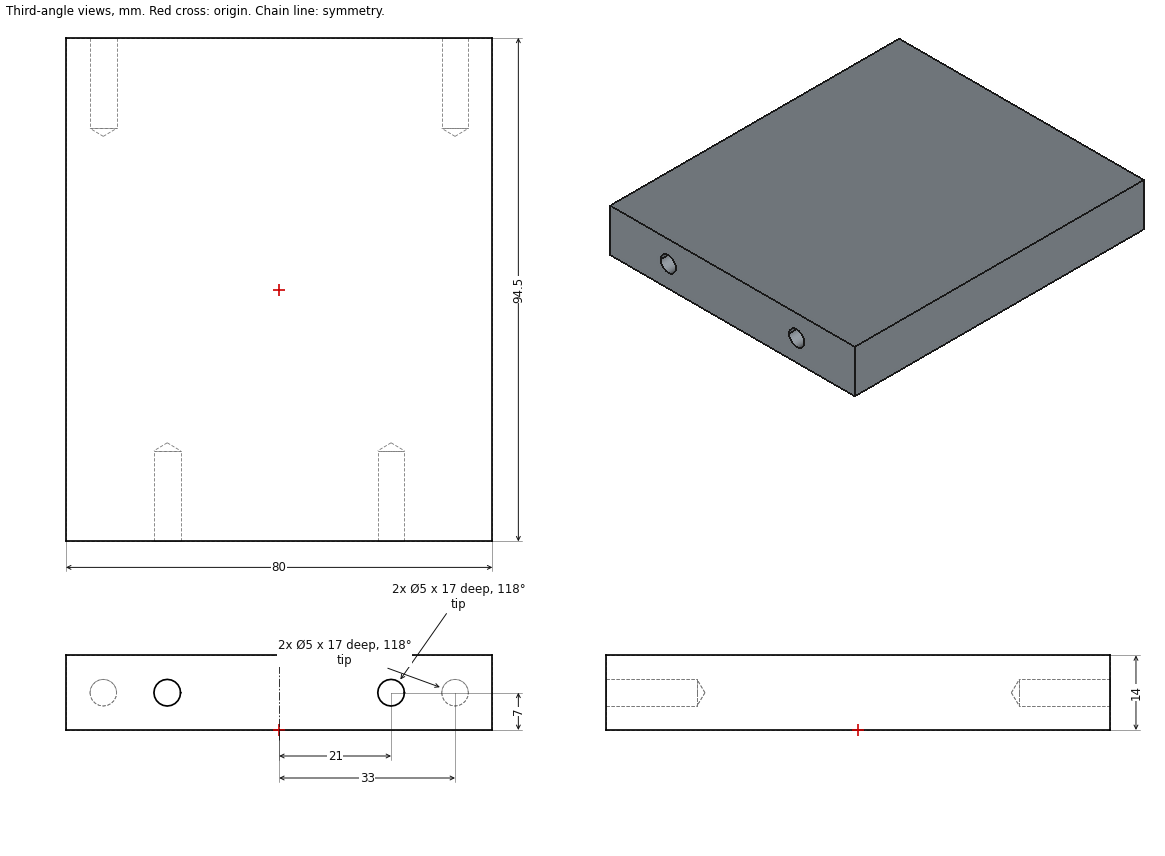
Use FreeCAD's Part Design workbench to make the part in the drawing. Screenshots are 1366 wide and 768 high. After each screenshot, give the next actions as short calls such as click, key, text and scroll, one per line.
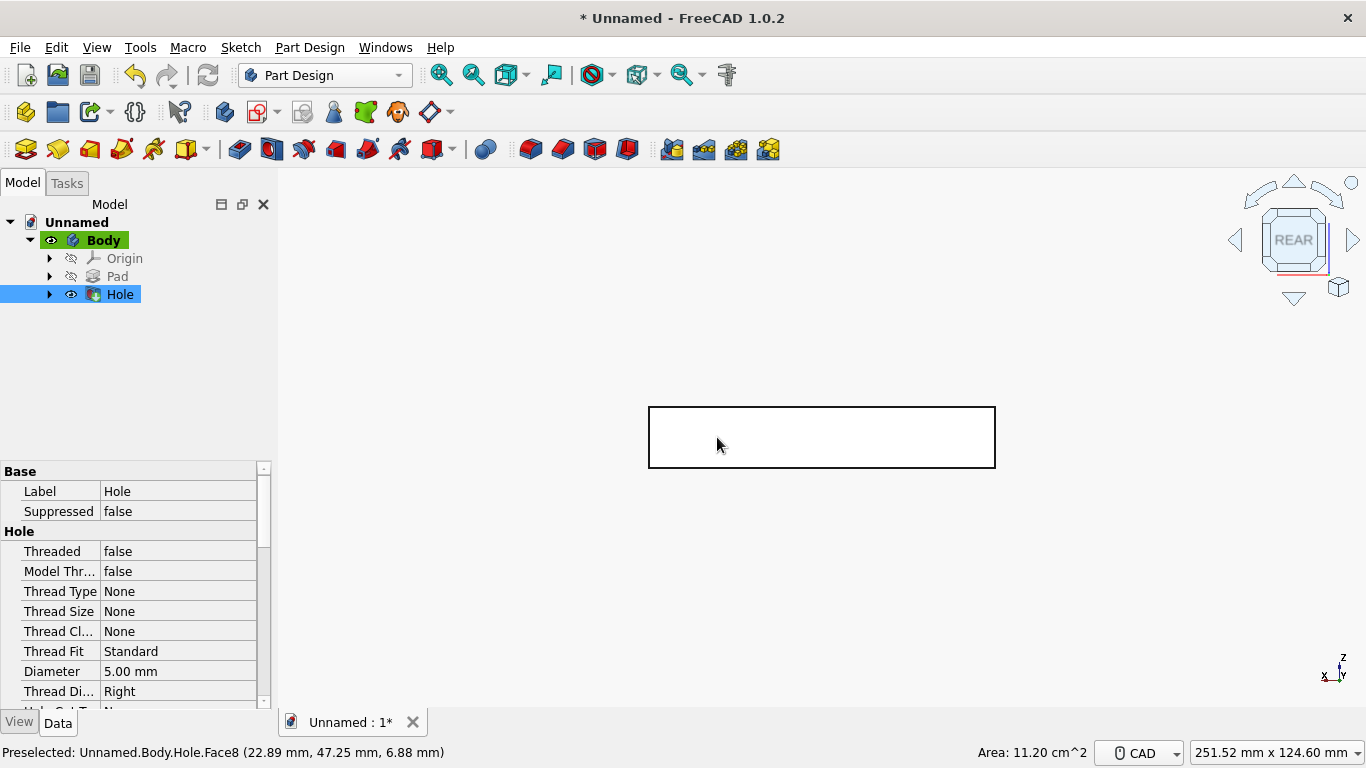
click(258, 112)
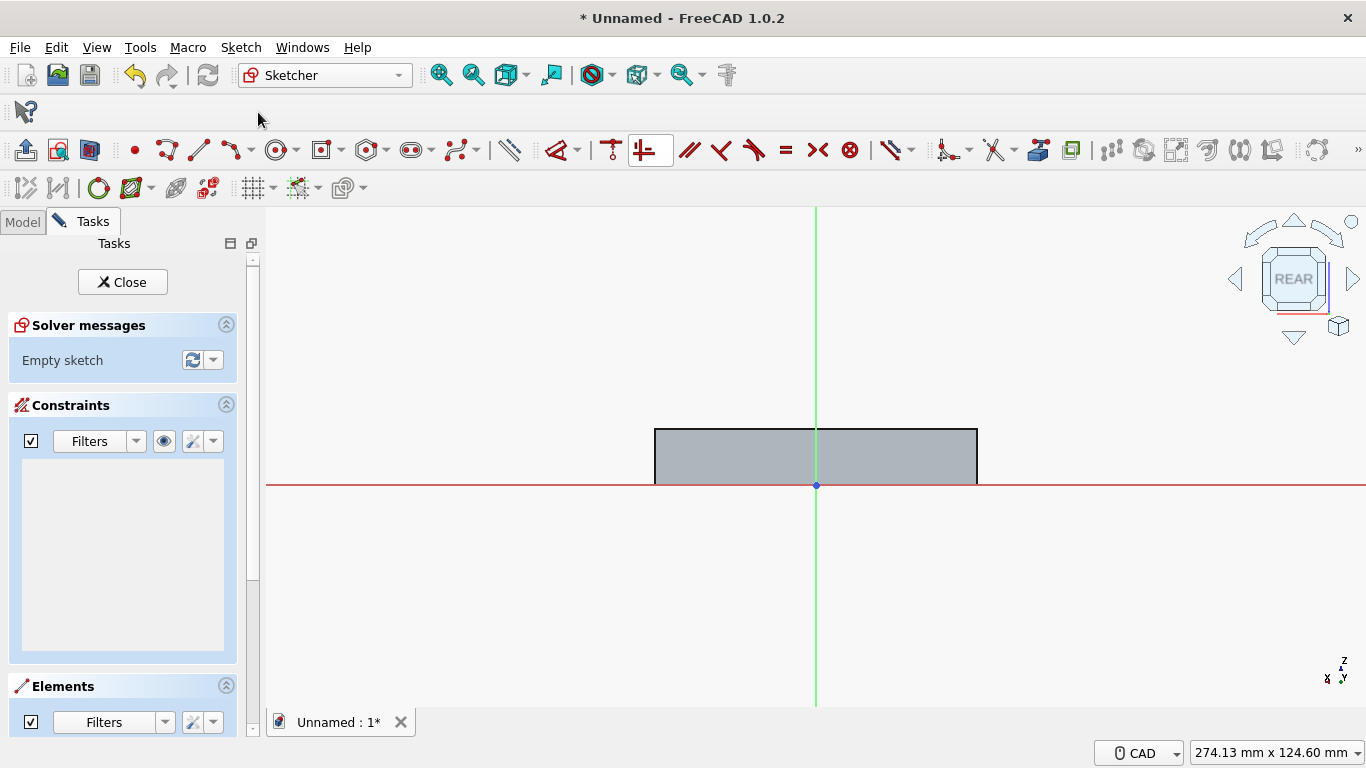
scroll(872, 473, up, 4)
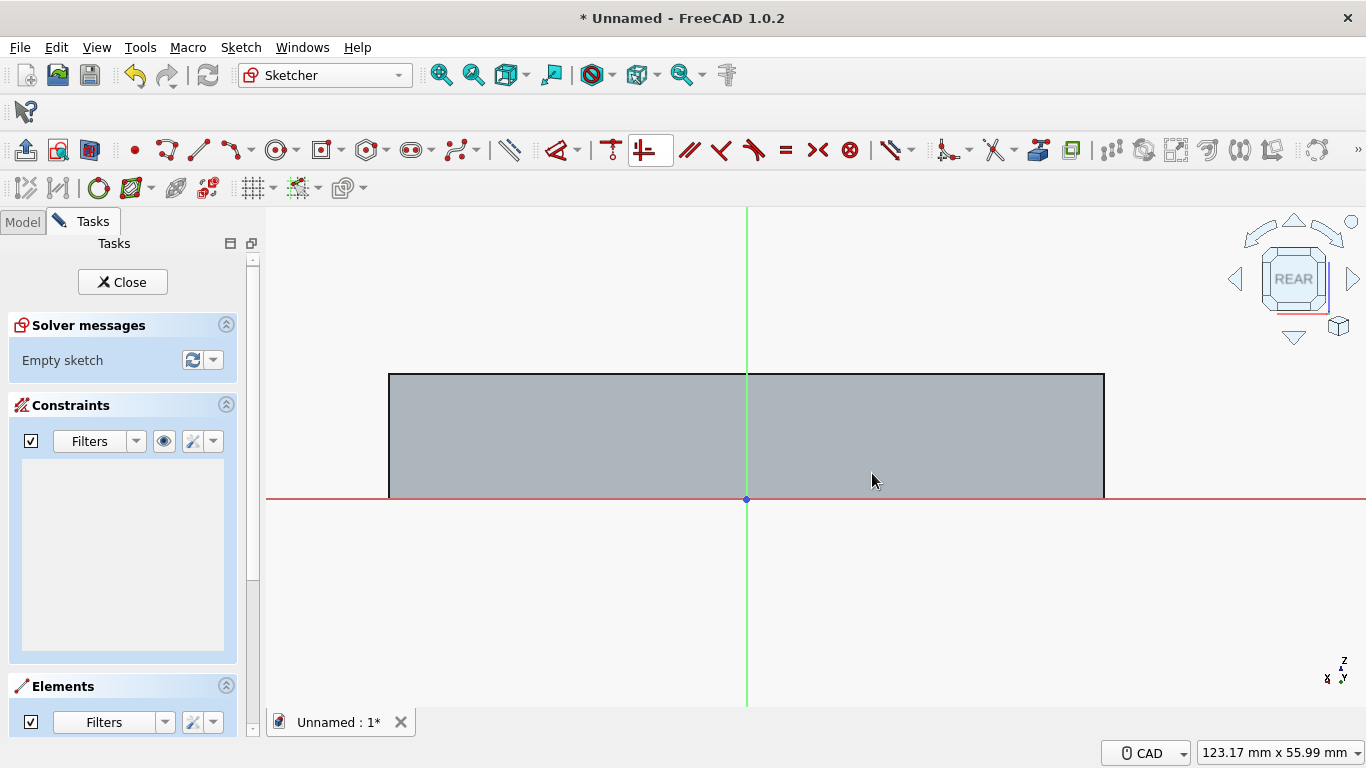
key(g)
key(c)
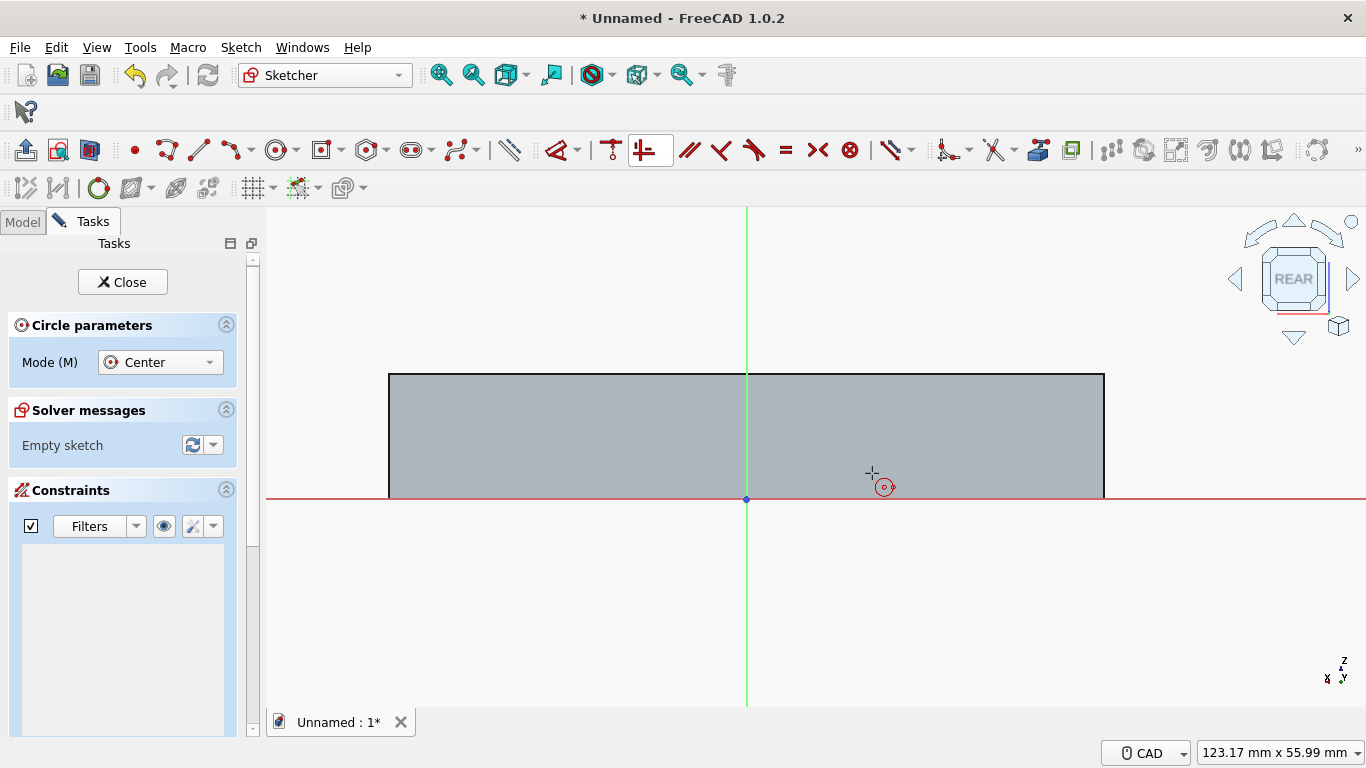
click(452, 437)
click(468, 421)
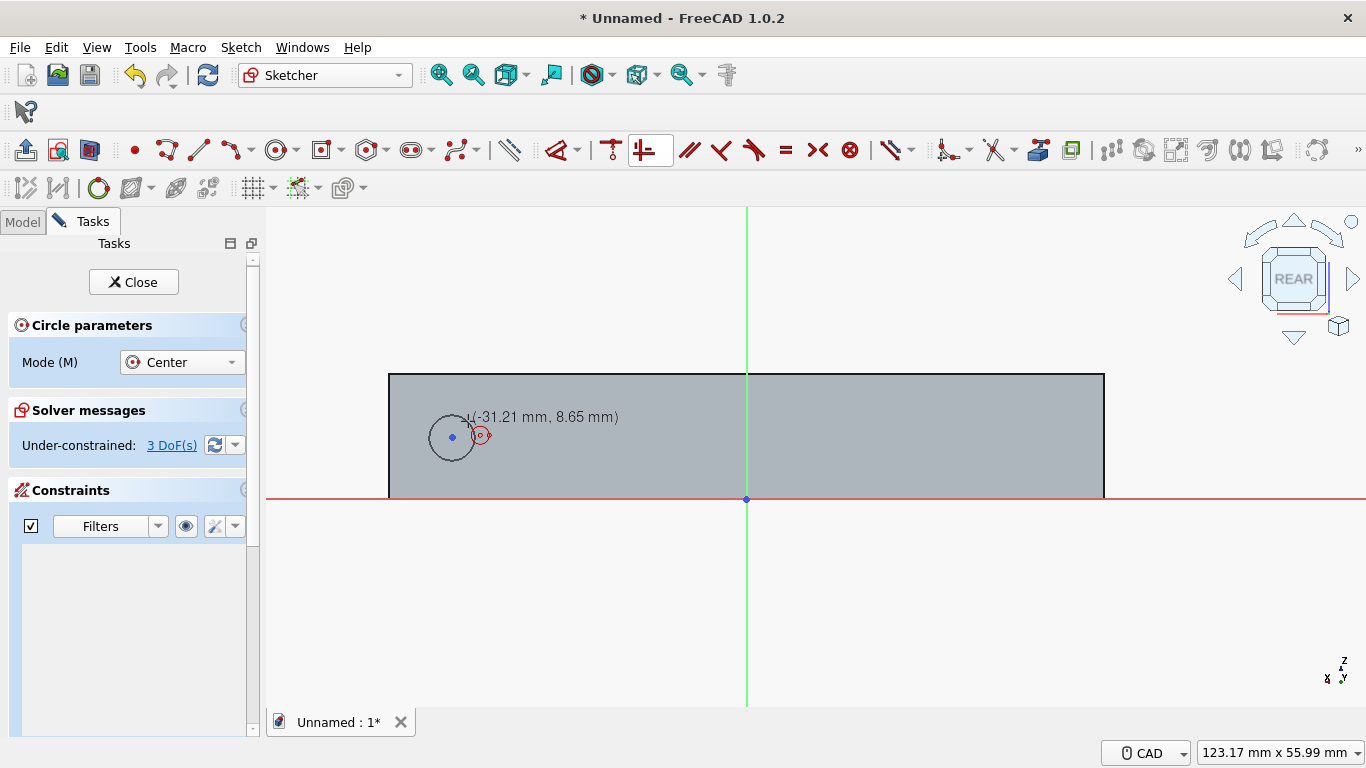
click(1041, 437)
click(1057, 421)
key(Escape)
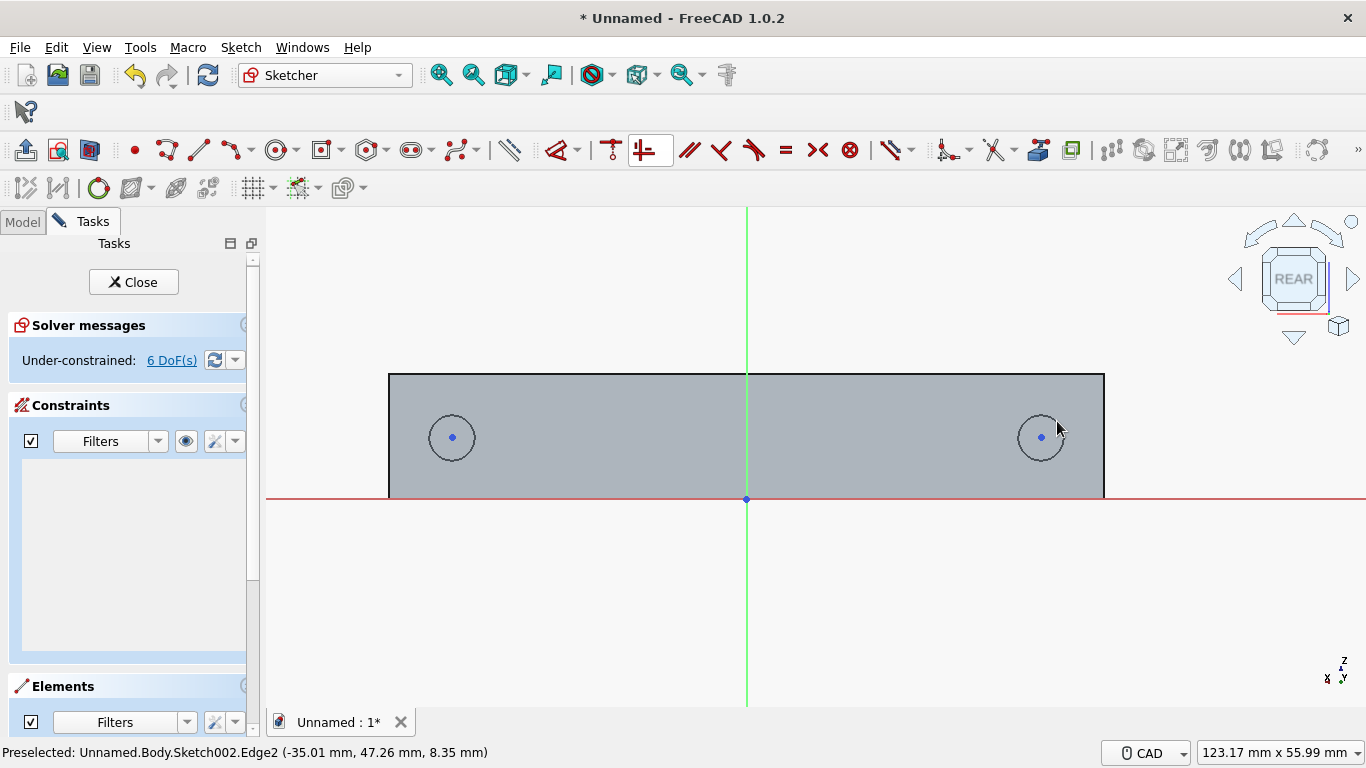
click(468, 422)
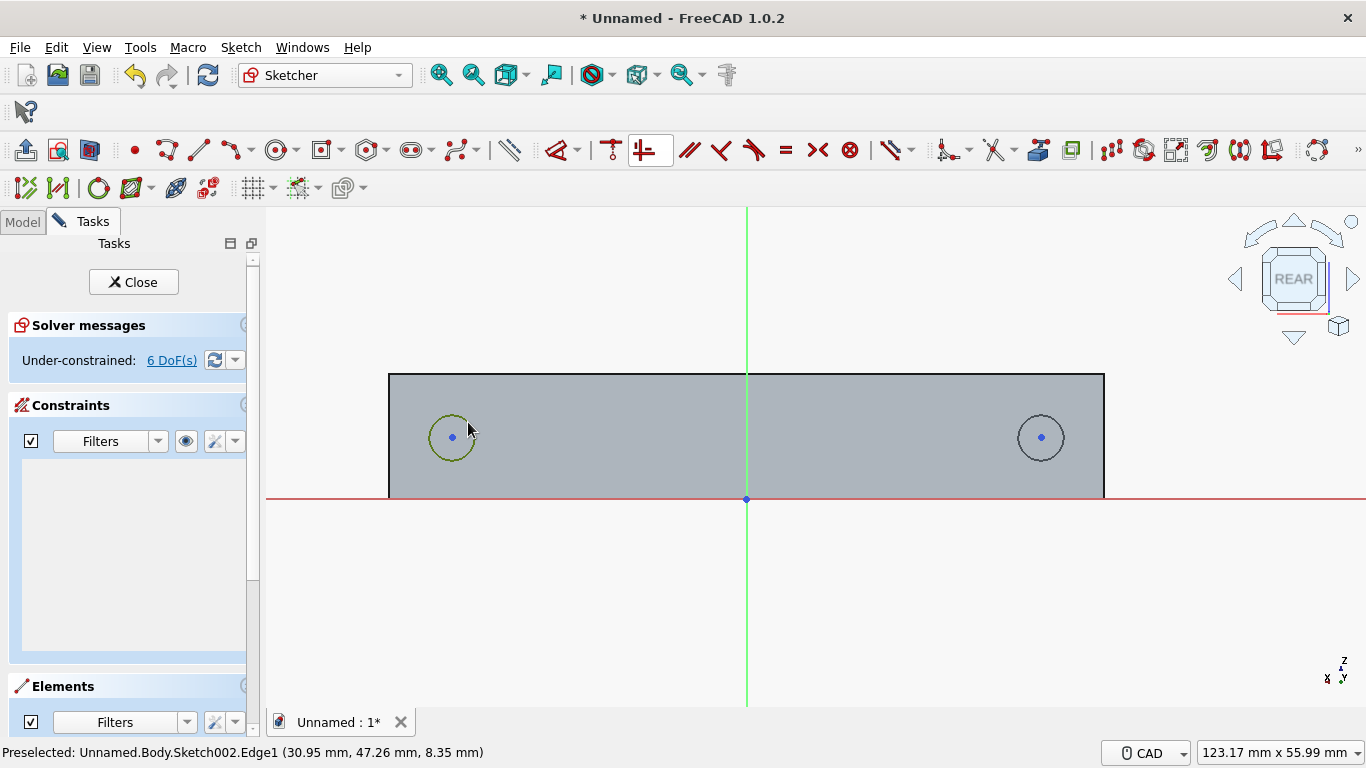
click(1057, 422)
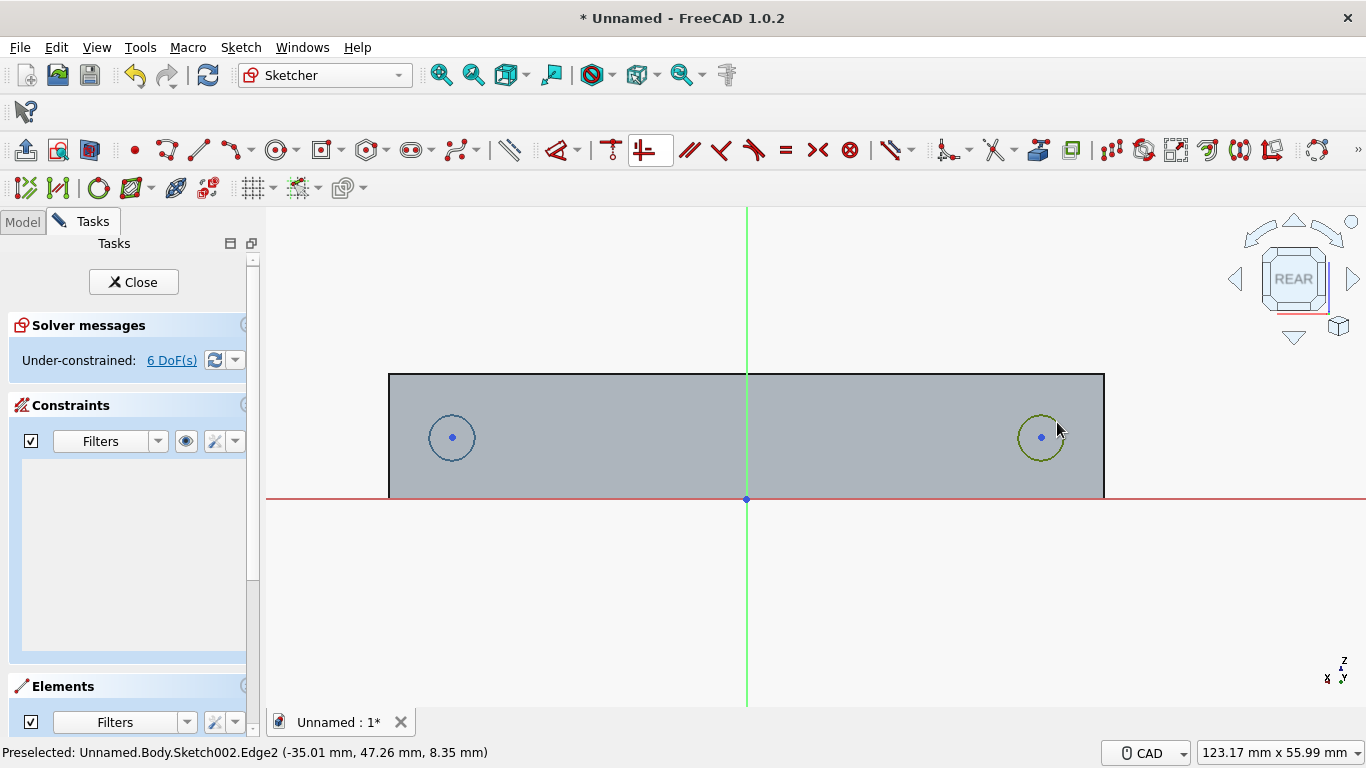
click(786, 150)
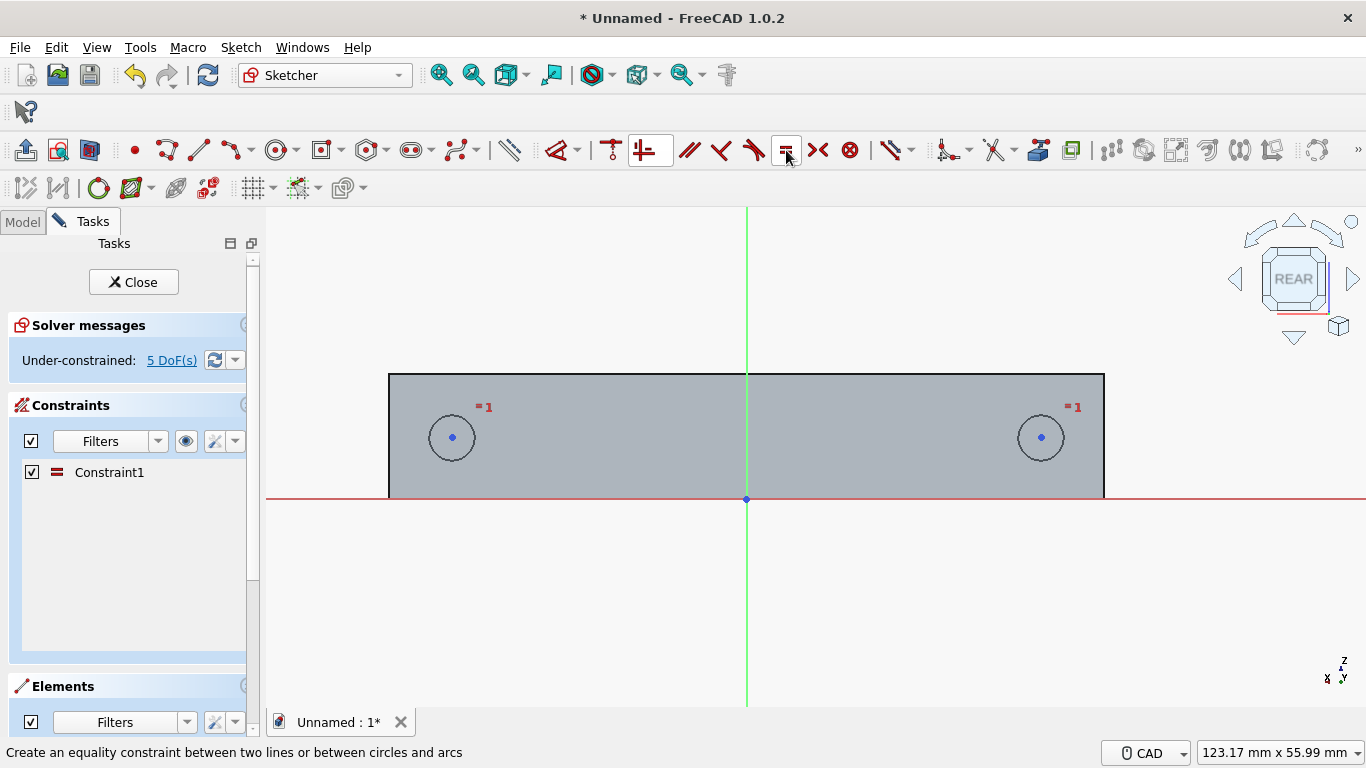
click(452, 438)